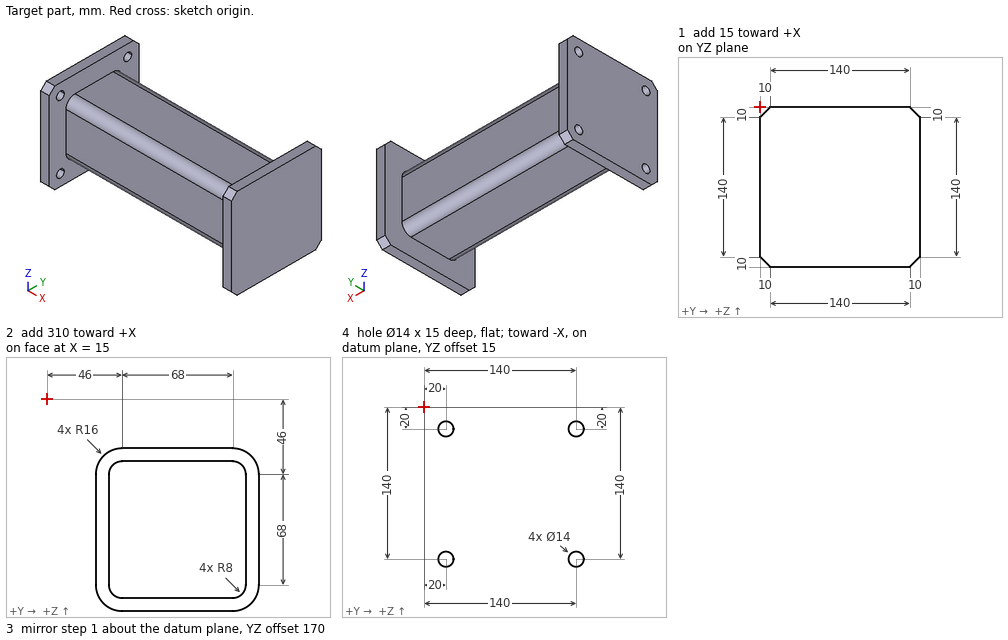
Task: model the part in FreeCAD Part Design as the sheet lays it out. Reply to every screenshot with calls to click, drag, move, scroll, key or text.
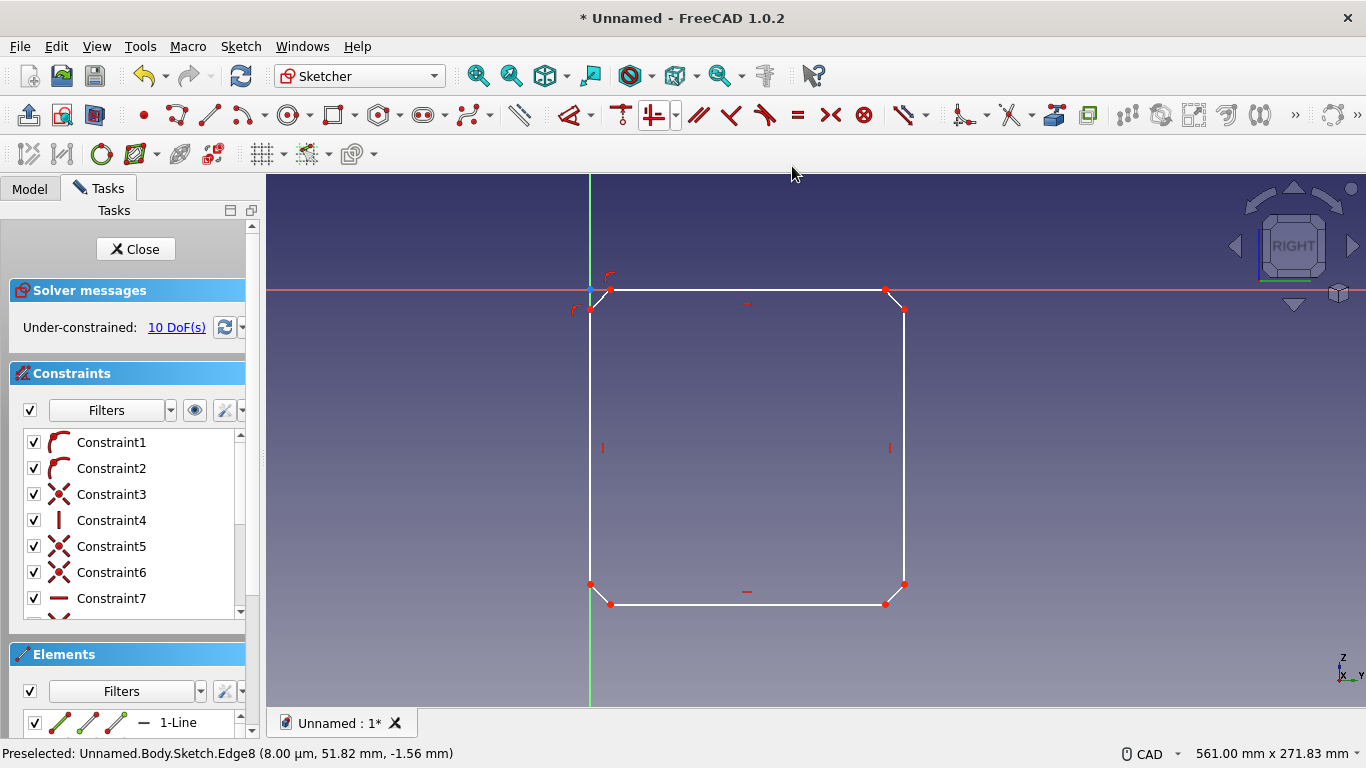
click(568, 116)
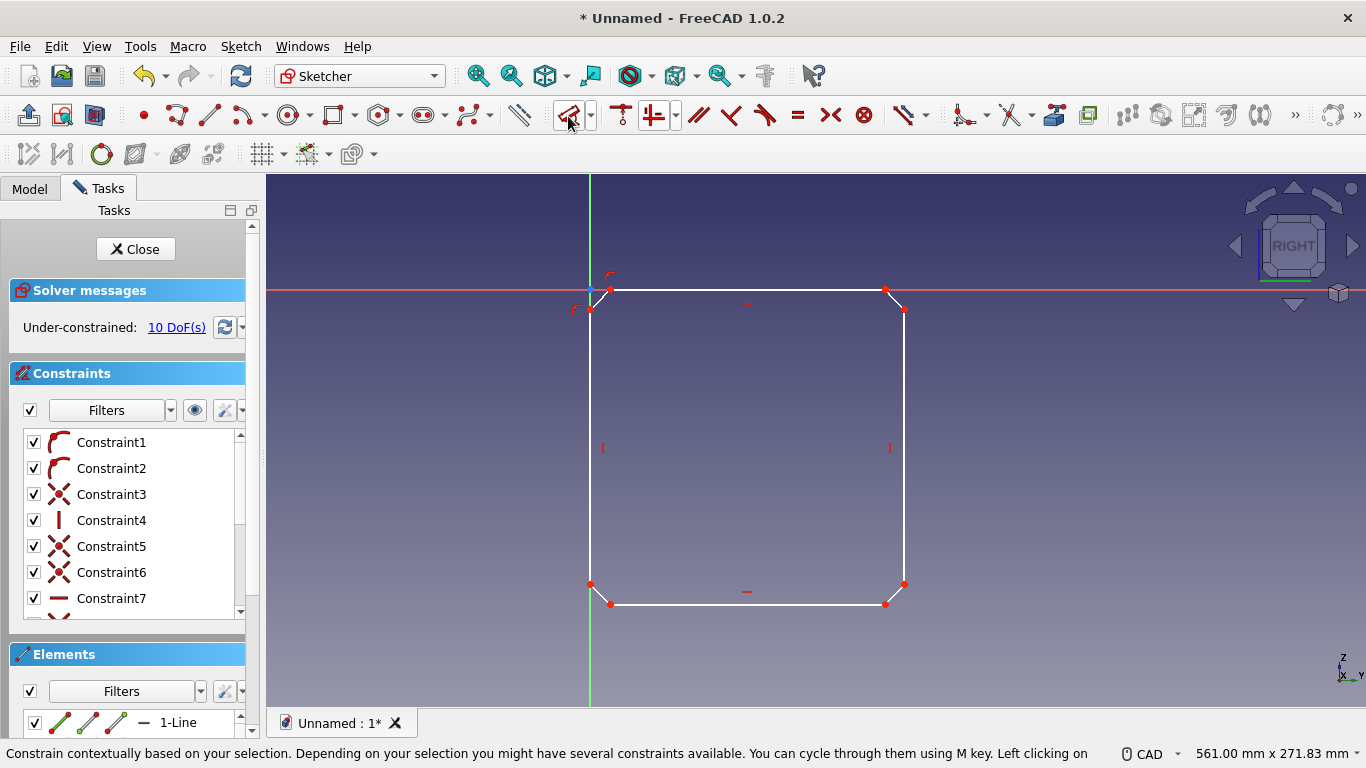
click(590, 393)
click(556, 448)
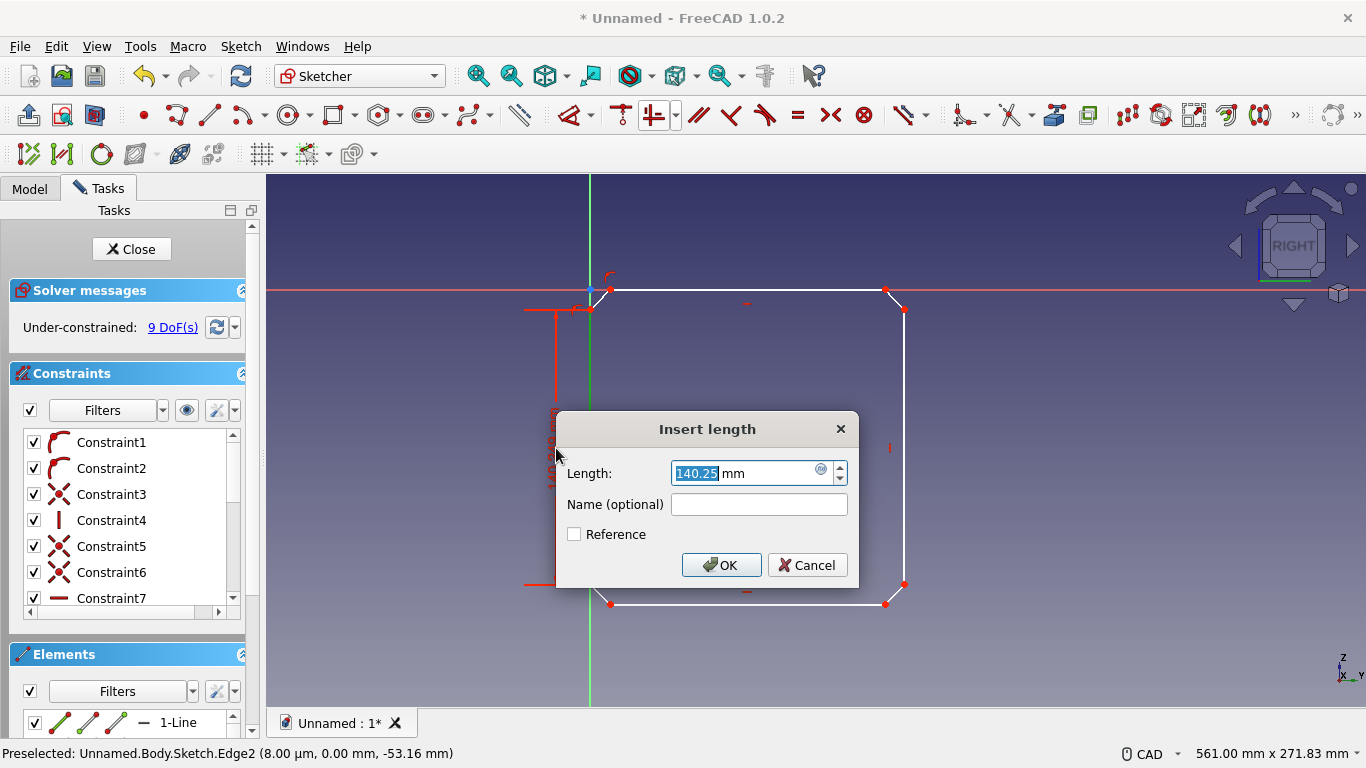
text(140)
key(Return)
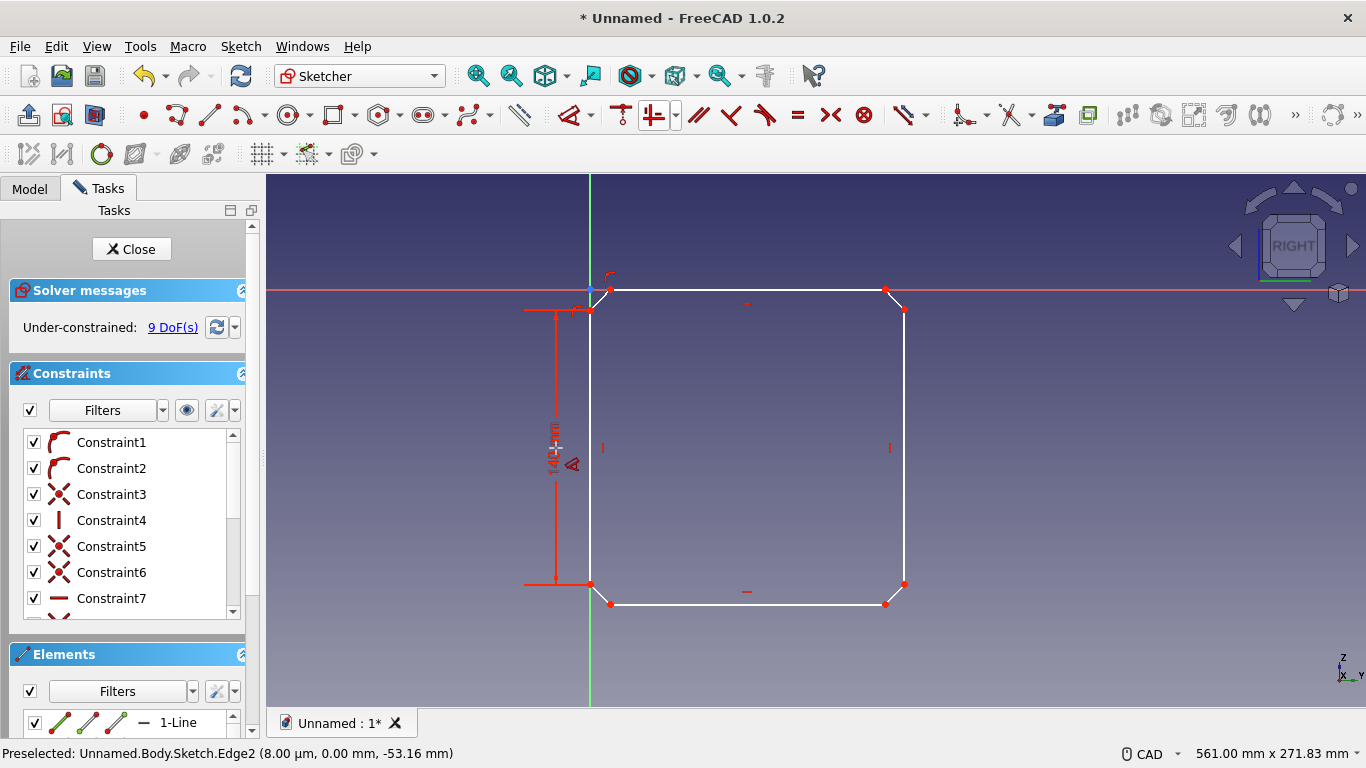
click(692, 605)
click(748, 639)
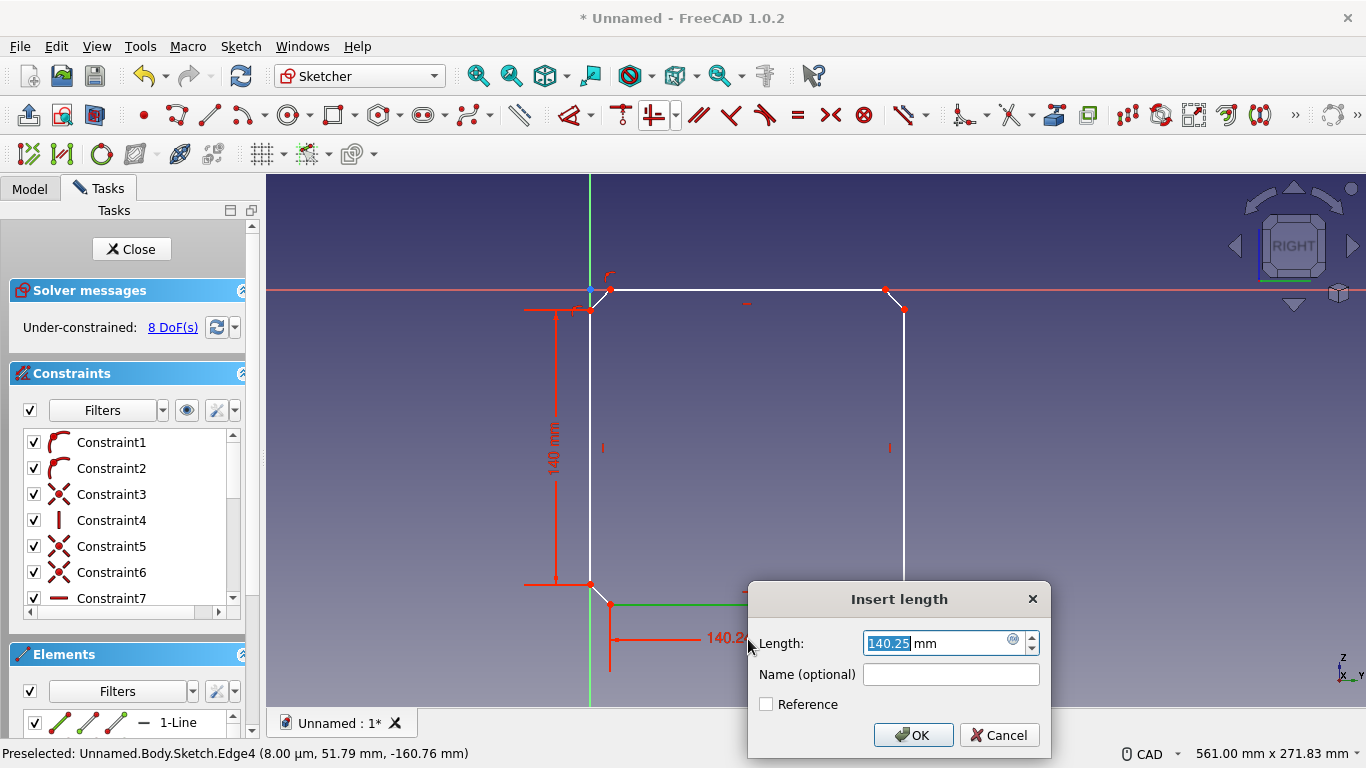
text(140)
key(Return)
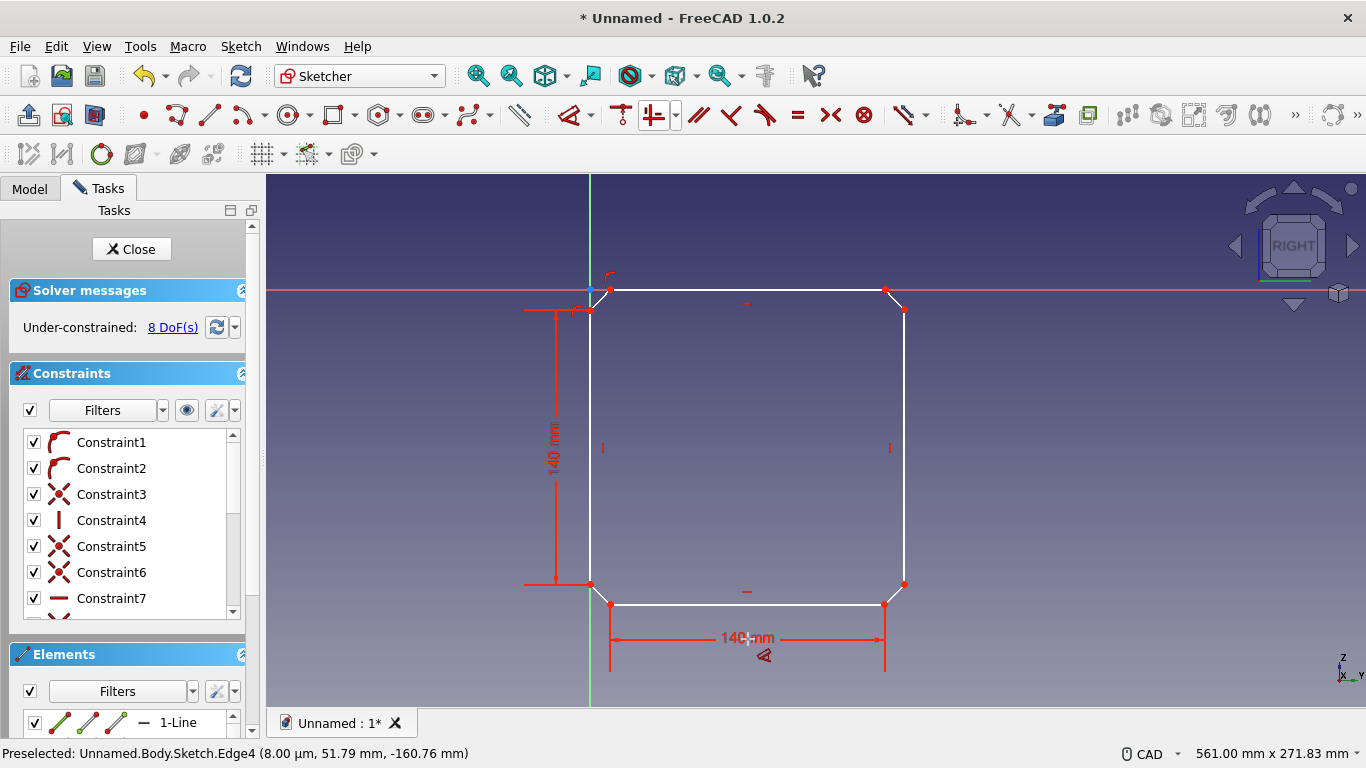
click(904, 503)
click(938, 448)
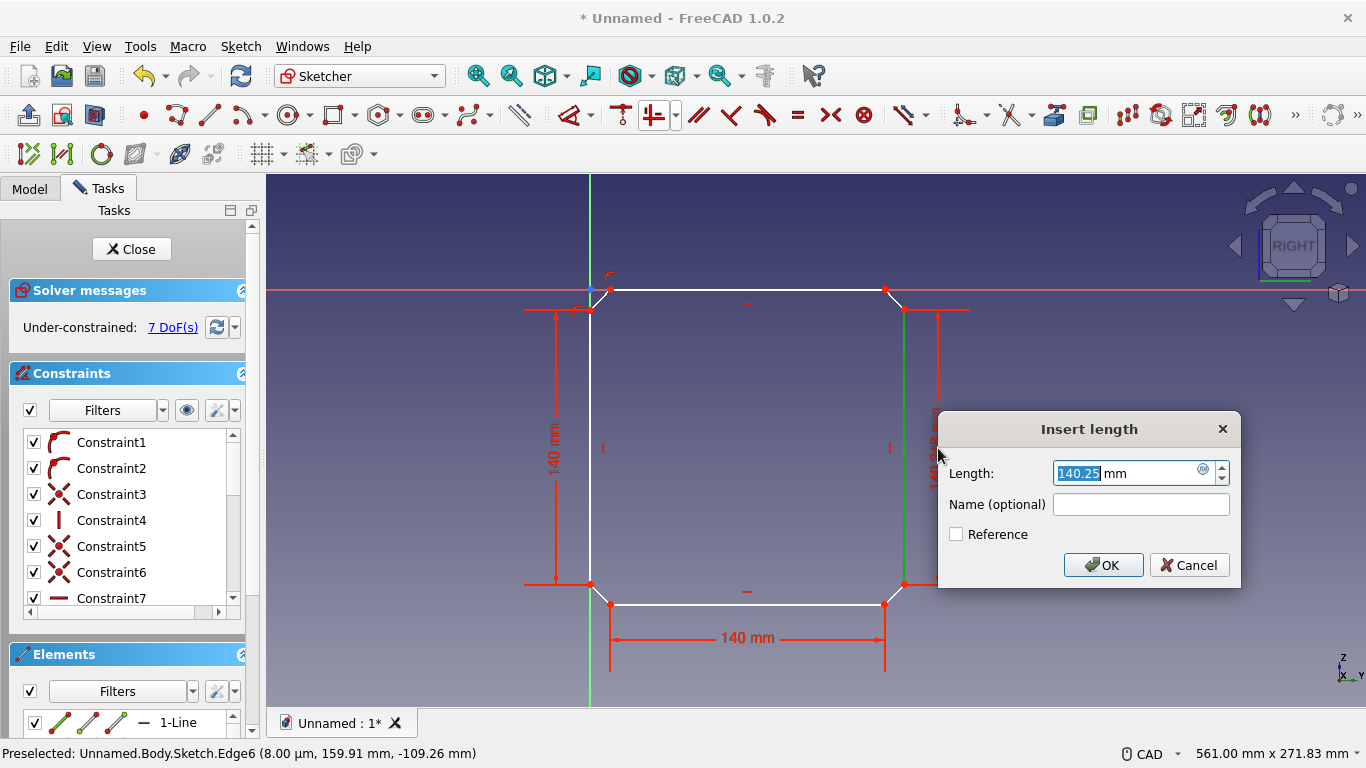
text(140)
key(Return)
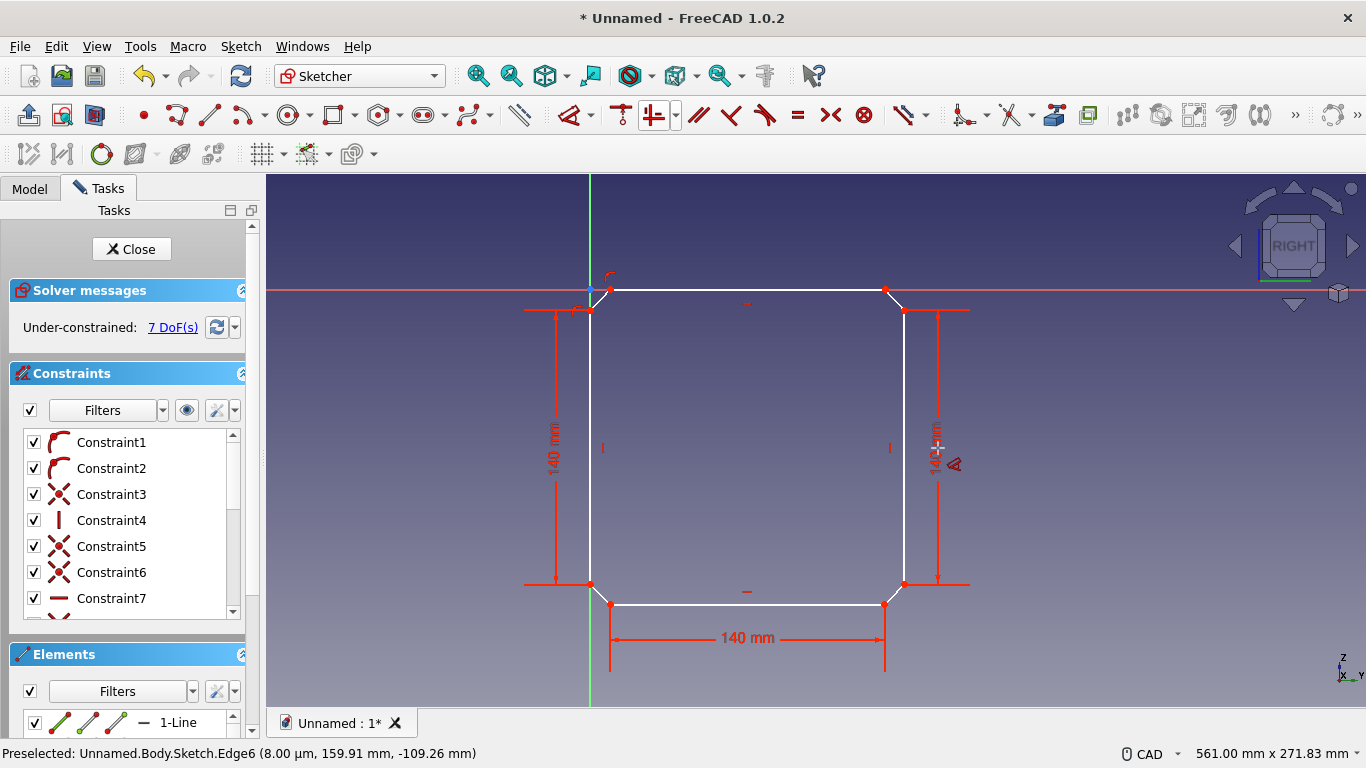
click(803, 290)
click(748, 256)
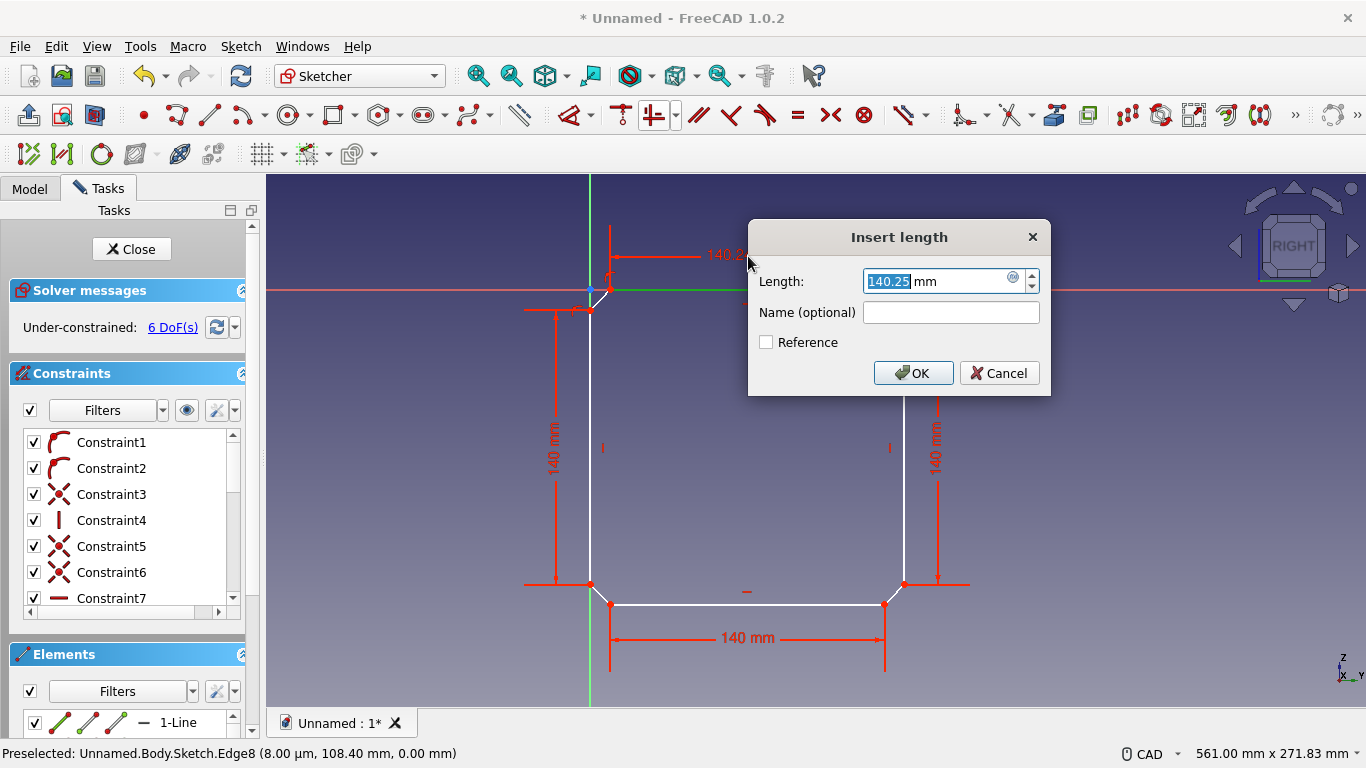
text(140)
key(Return)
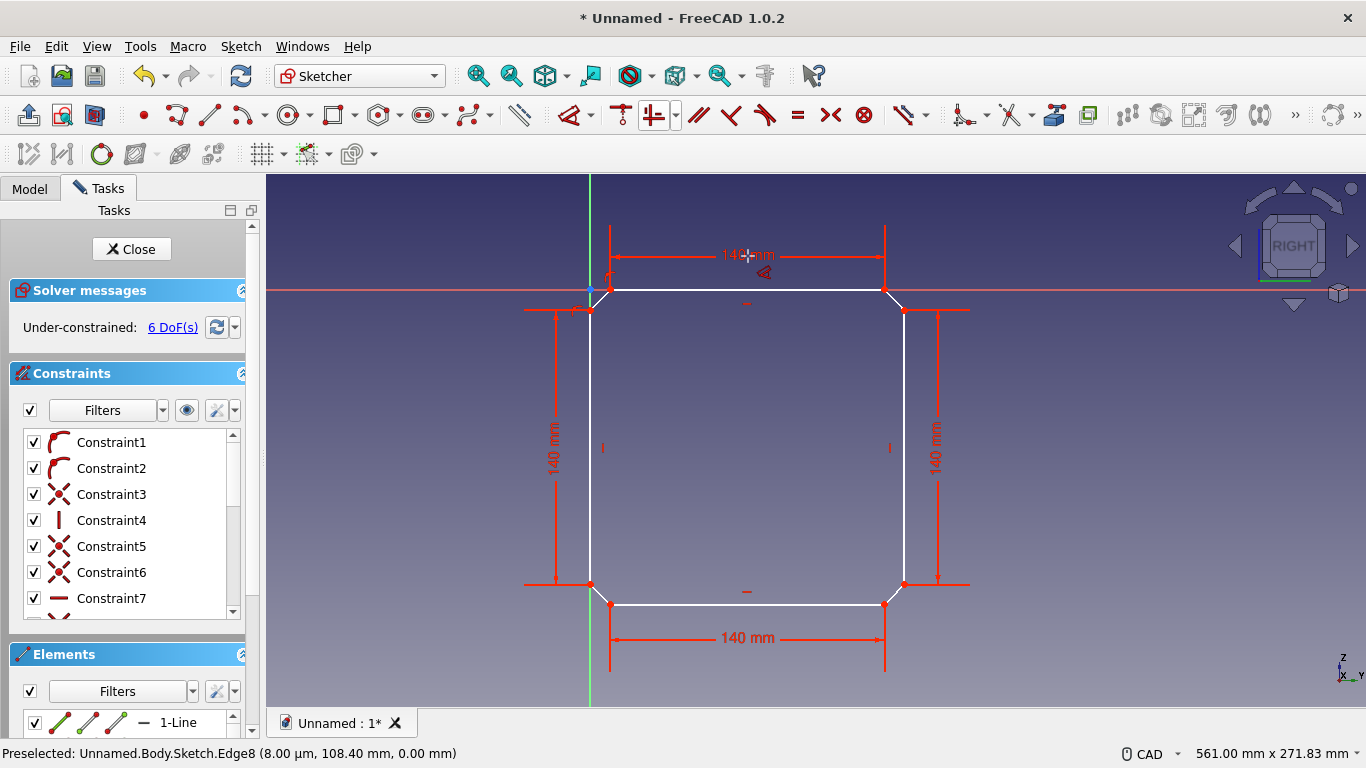
scroll(610, 290, up, 4)